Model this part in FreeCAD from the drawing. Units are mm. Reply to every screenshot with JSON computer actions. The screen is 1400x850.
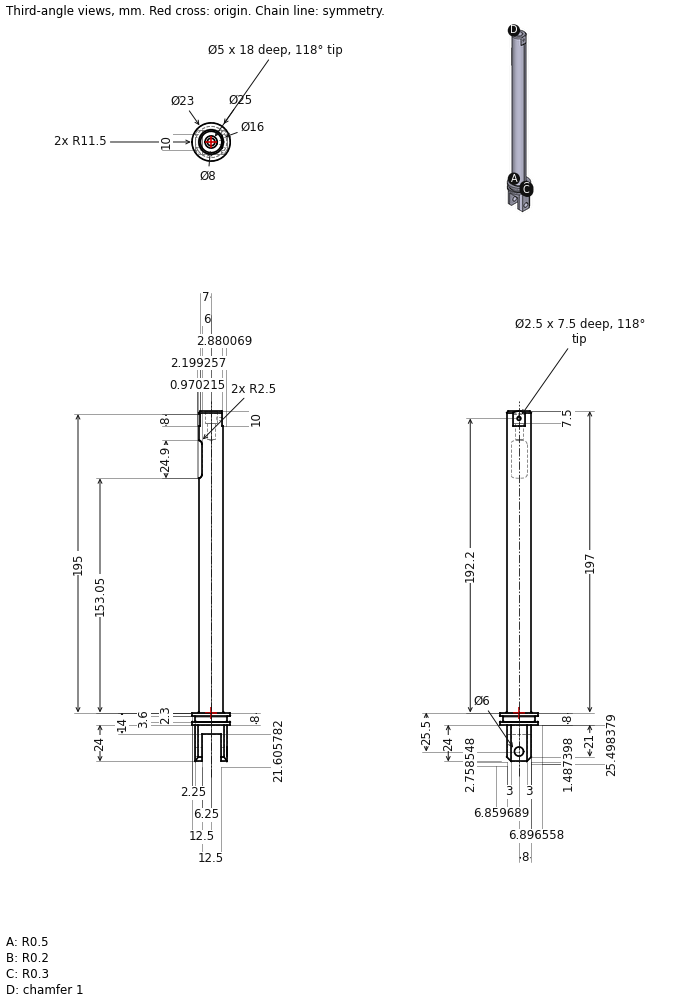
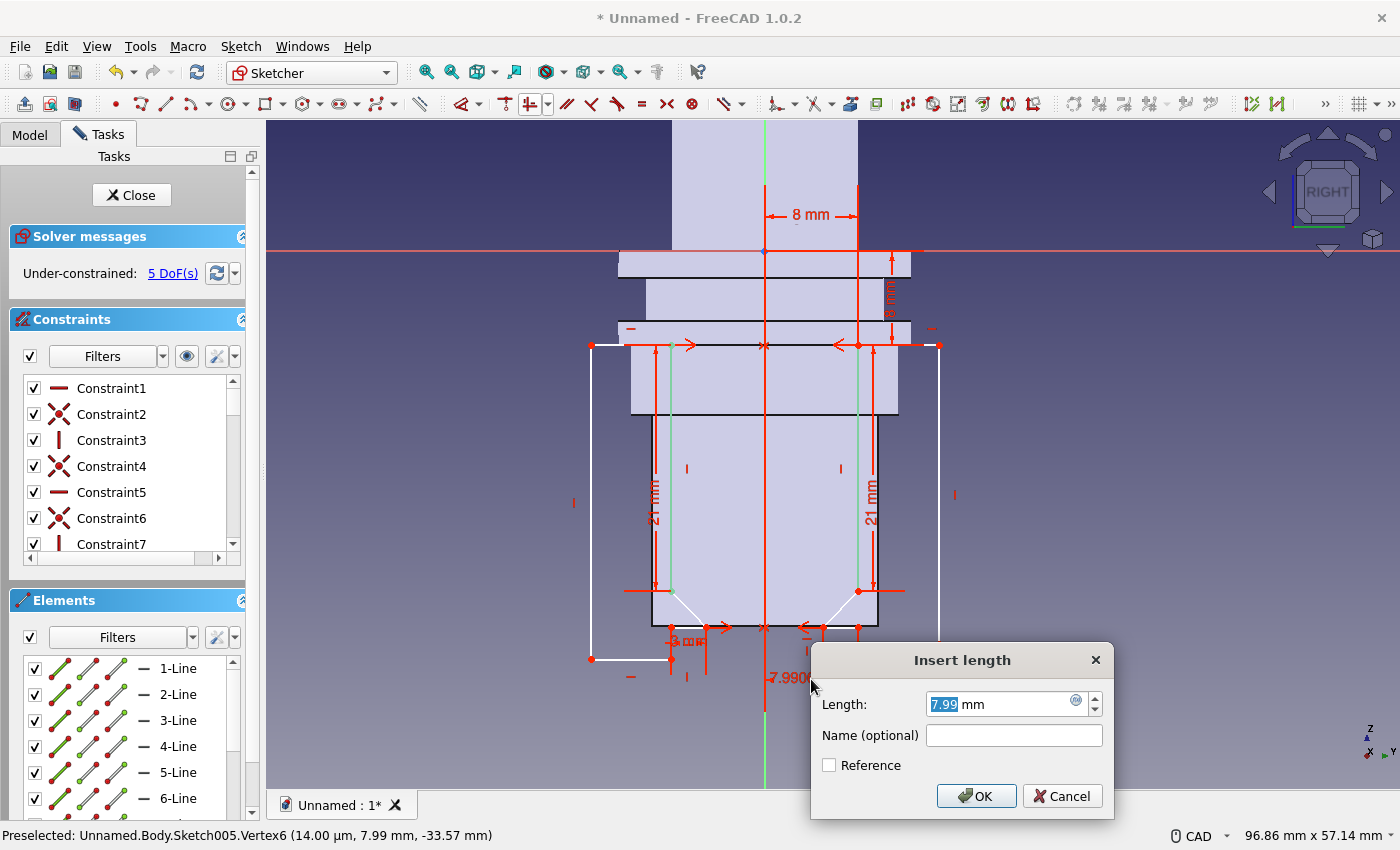
{"action": "type", "text": "8"}
{"action": "key", "text": "Return"}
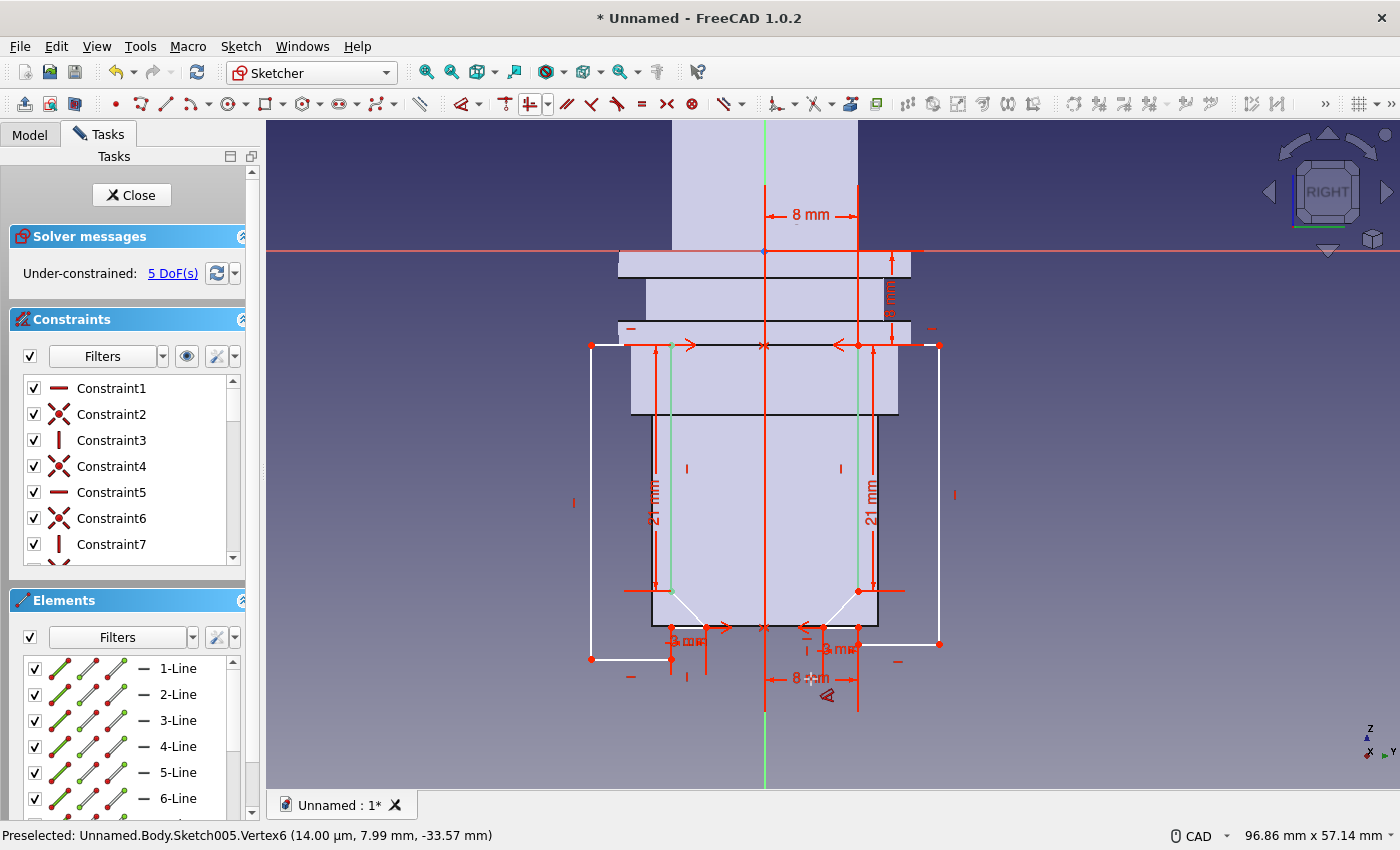
{"action": "left_click", "coordinate": [883, 345]}
{"action": "left_click", "coordinate": [899, 379]}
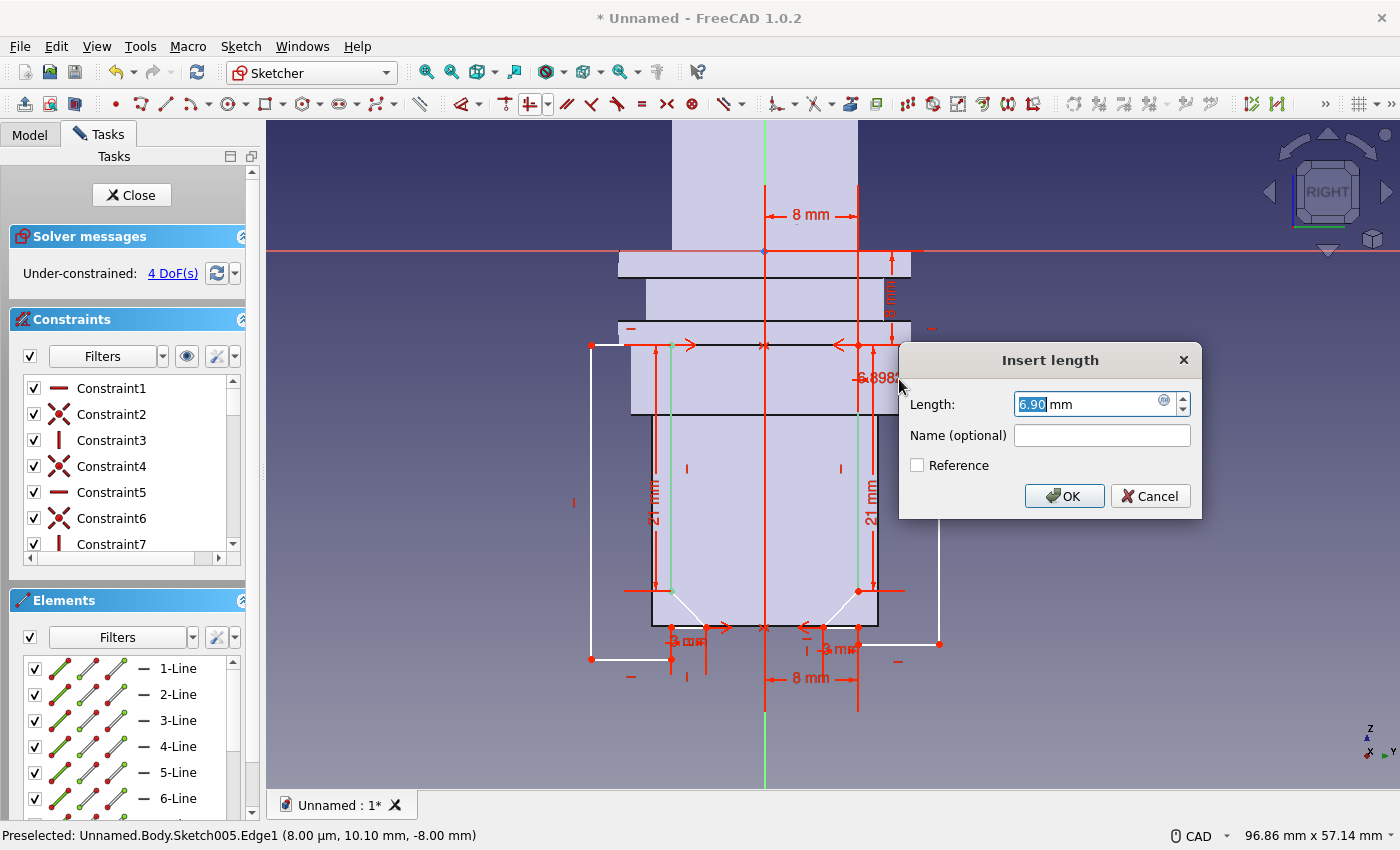
{"action": "type", "text": "6.896558"}
{"action": "key", "text": "Return"}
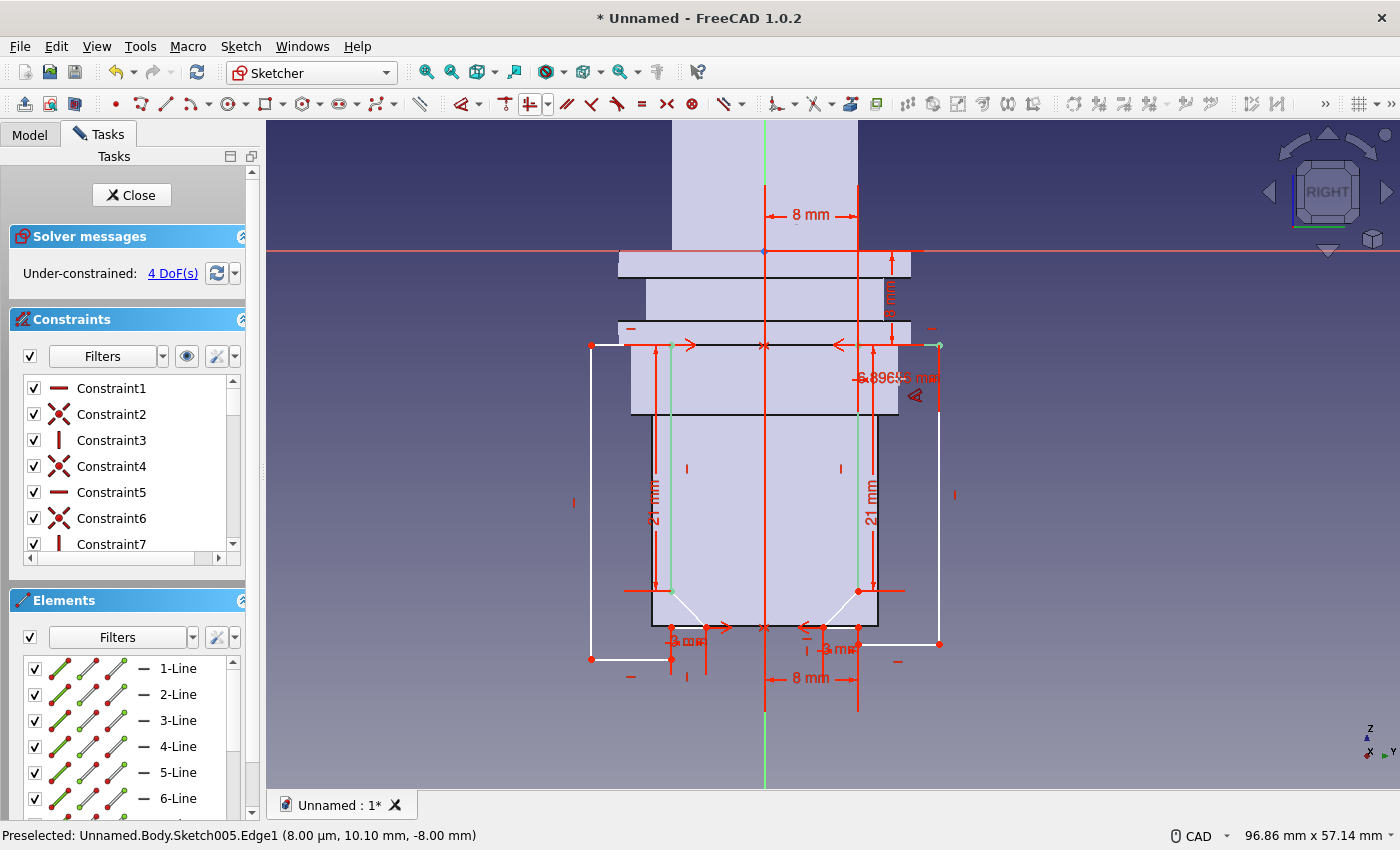
{"action": "scroll", "coordinate": [858, 636], "scroll_direction": "up", "scroll_amount": 5}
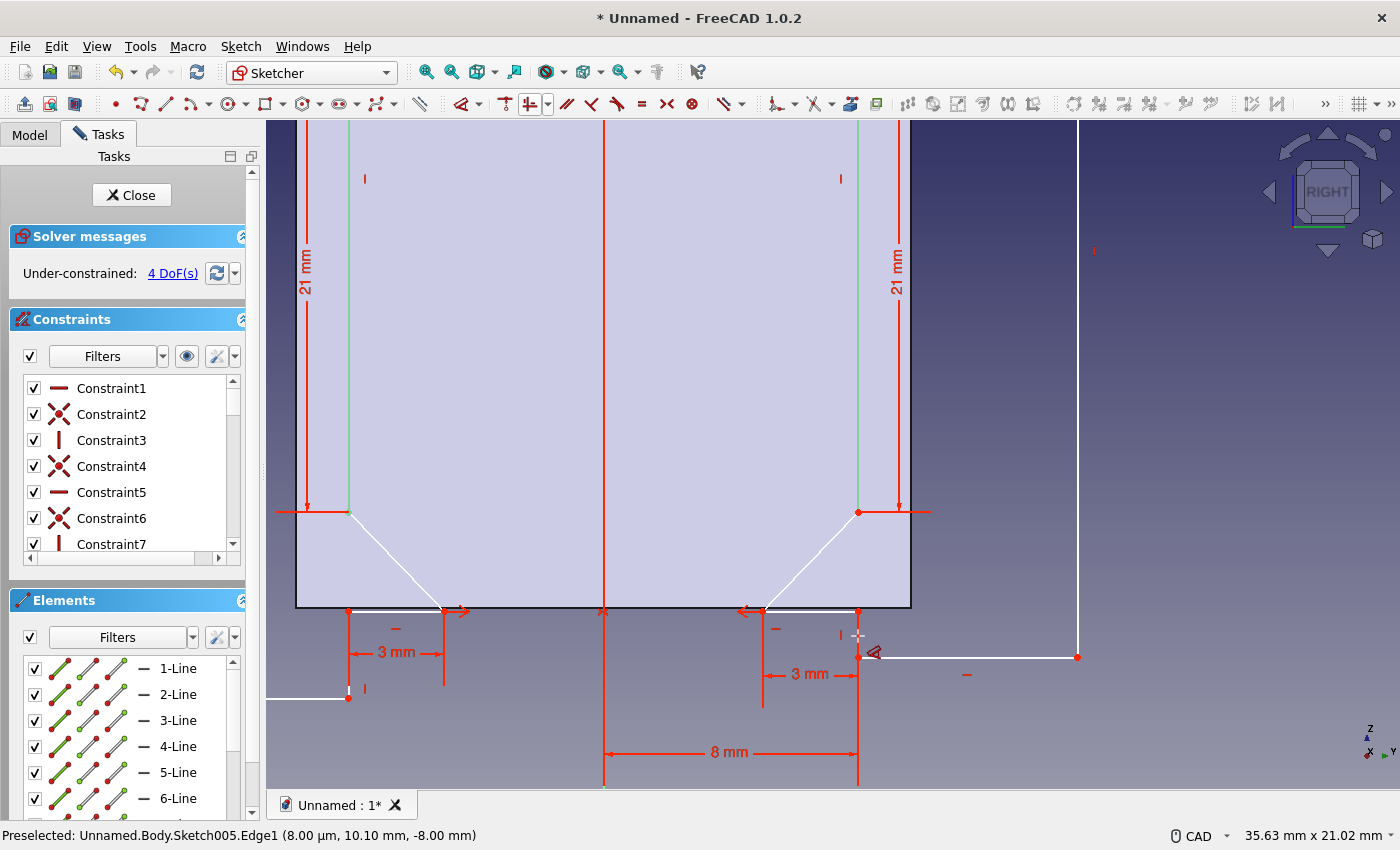
{"action": "left_click", "coordinate": [858, 635]}
{"action": "left_click", "coordinate": [892, 635]}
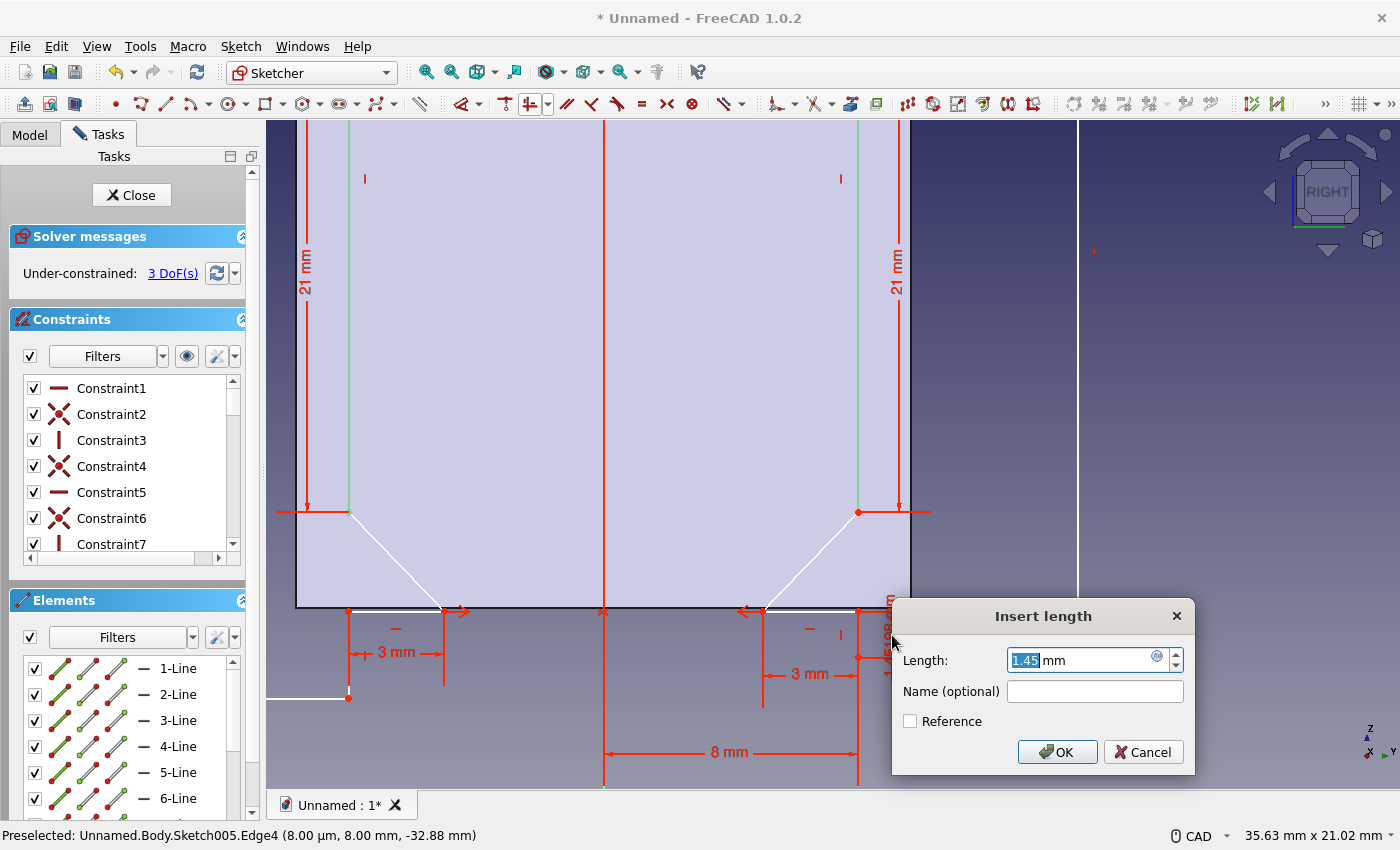
{"action": "type", "text": "1.487398"}
{"action": "key", "text": "Return"}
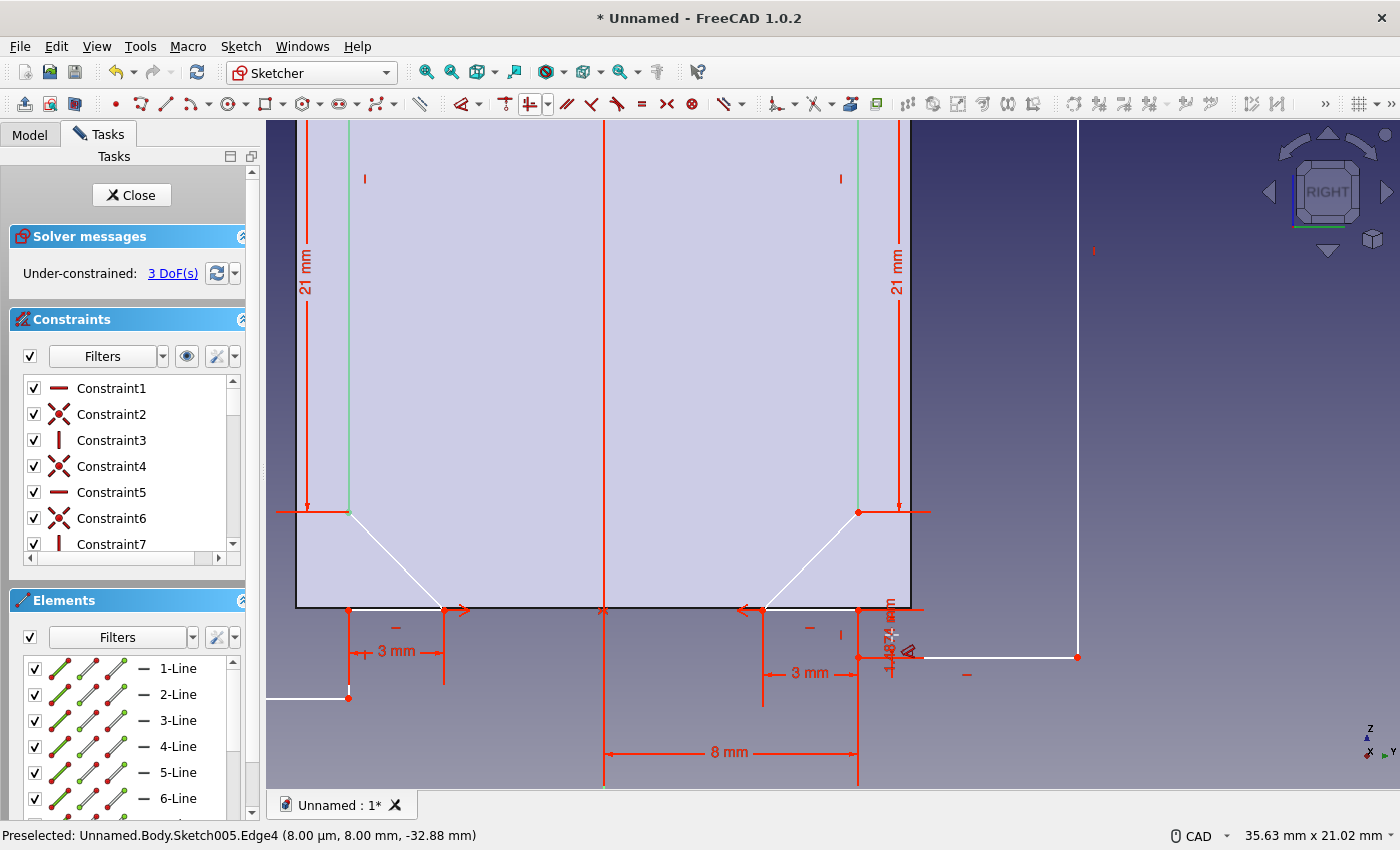
{"action": "left_click", "coordinate": [349, 637]}
{"action": "left_click", "coordinate": [315, 655]}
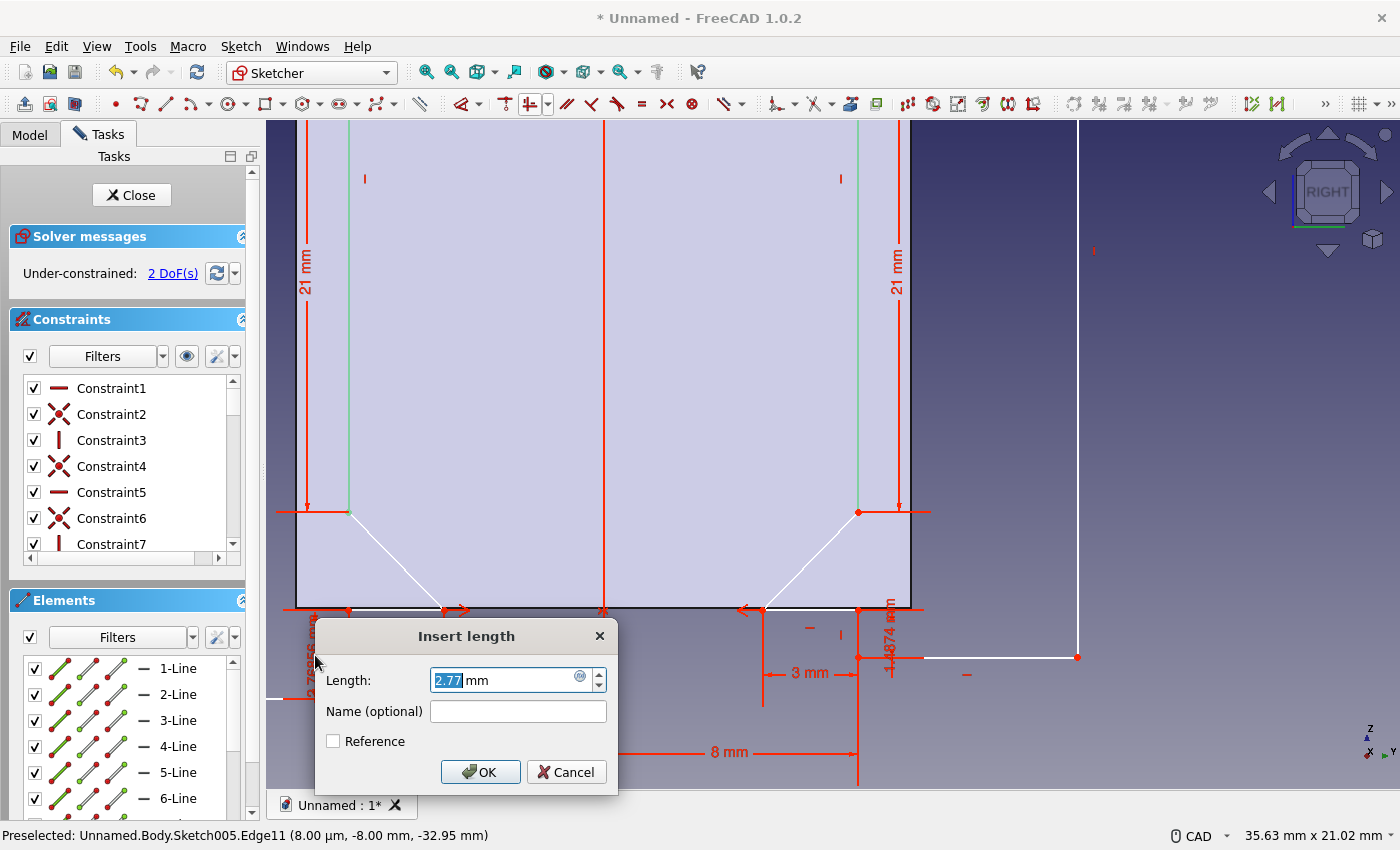
{"action": "type", "text": "2.758548"}
{"action": "key", "text": "Return"}